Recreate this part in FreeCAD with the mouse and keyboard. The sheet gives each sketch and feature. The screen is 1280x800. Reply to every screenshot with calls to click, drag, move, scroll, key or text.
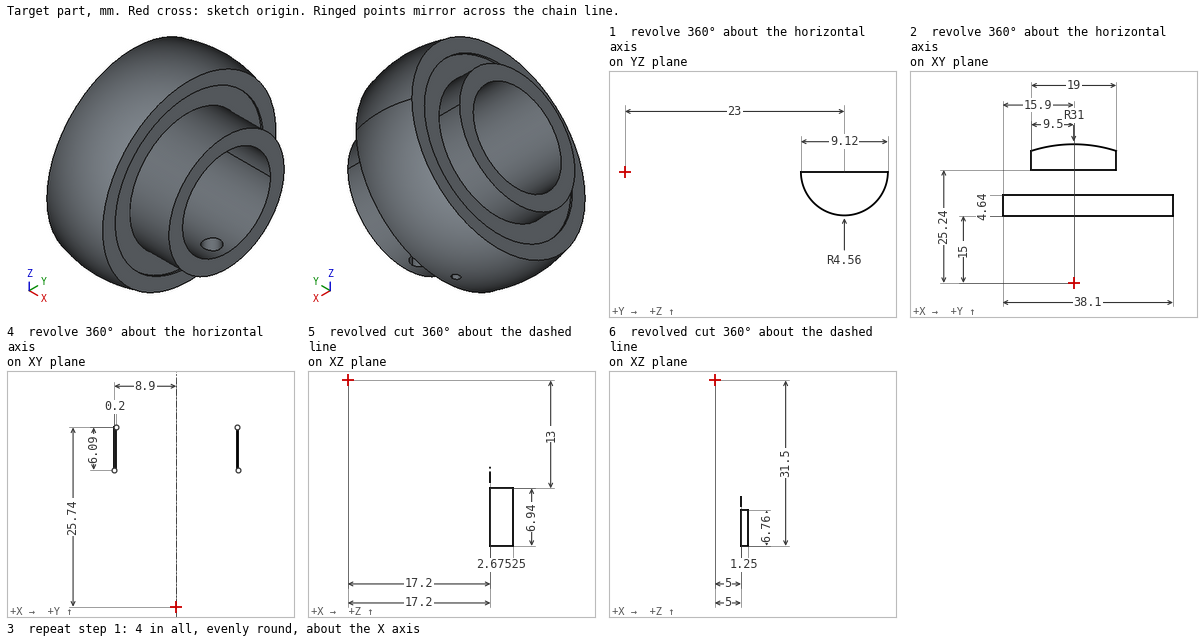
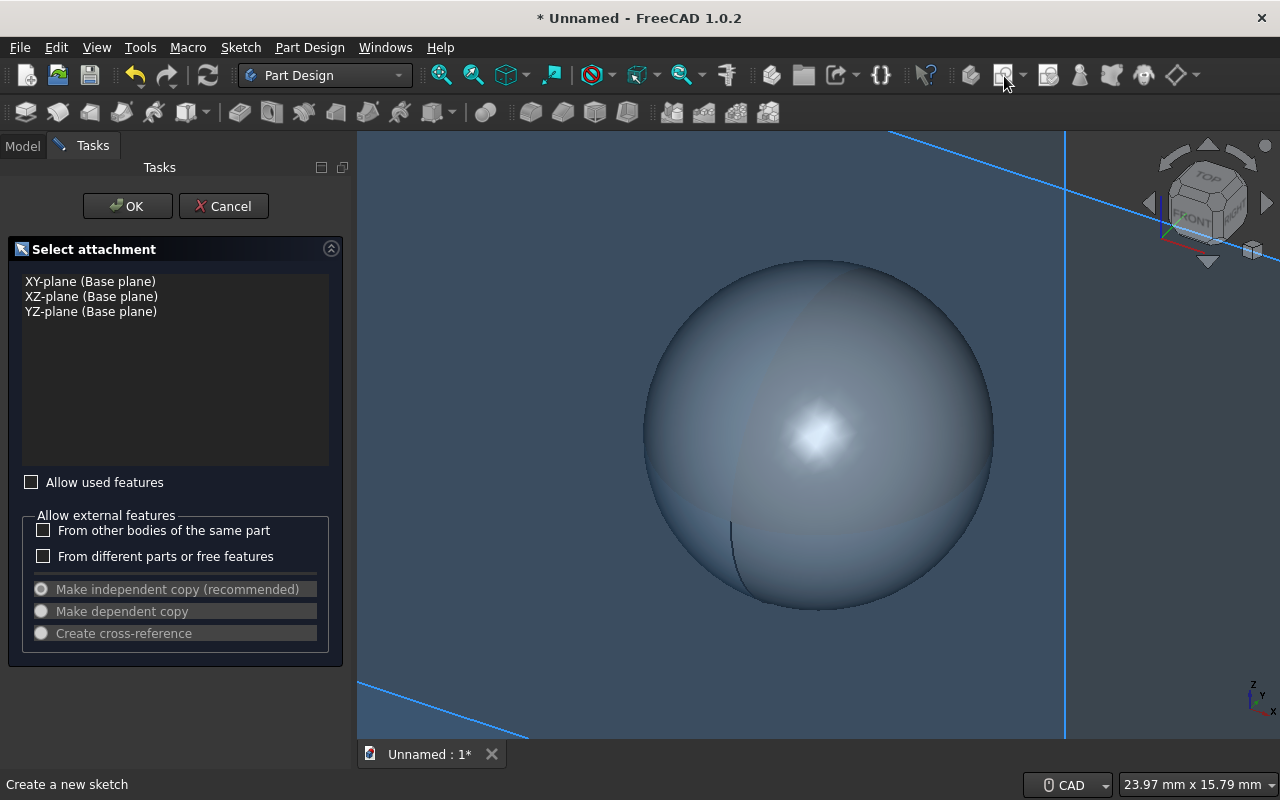
click(82, 282)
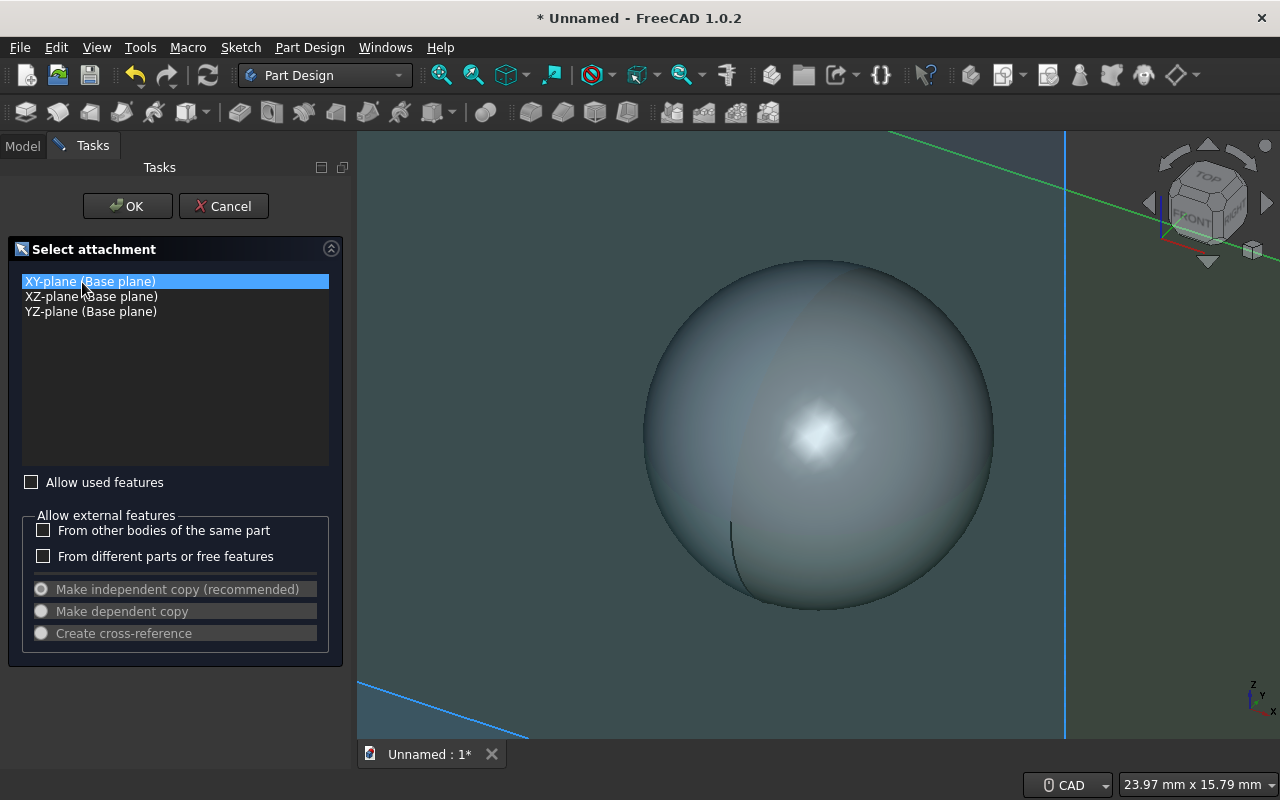
click(128, 206)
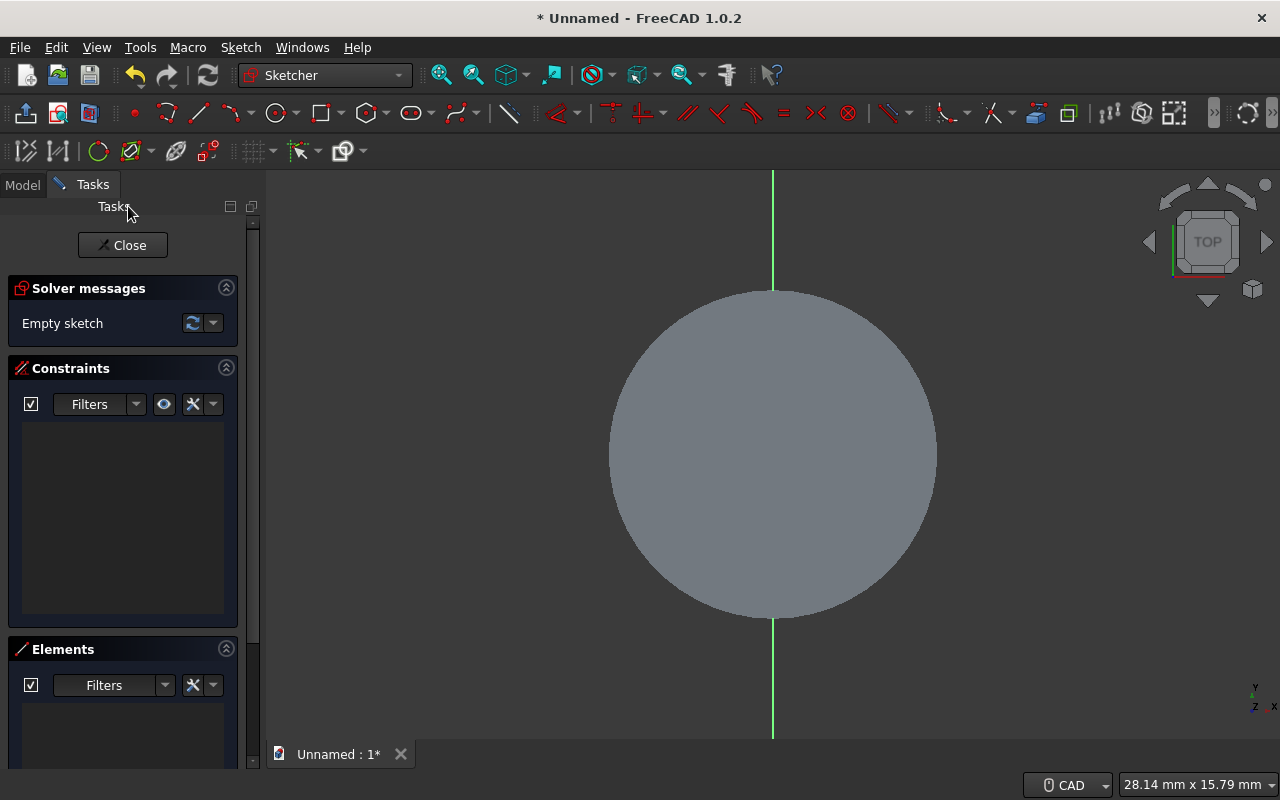
key(q)
key(s)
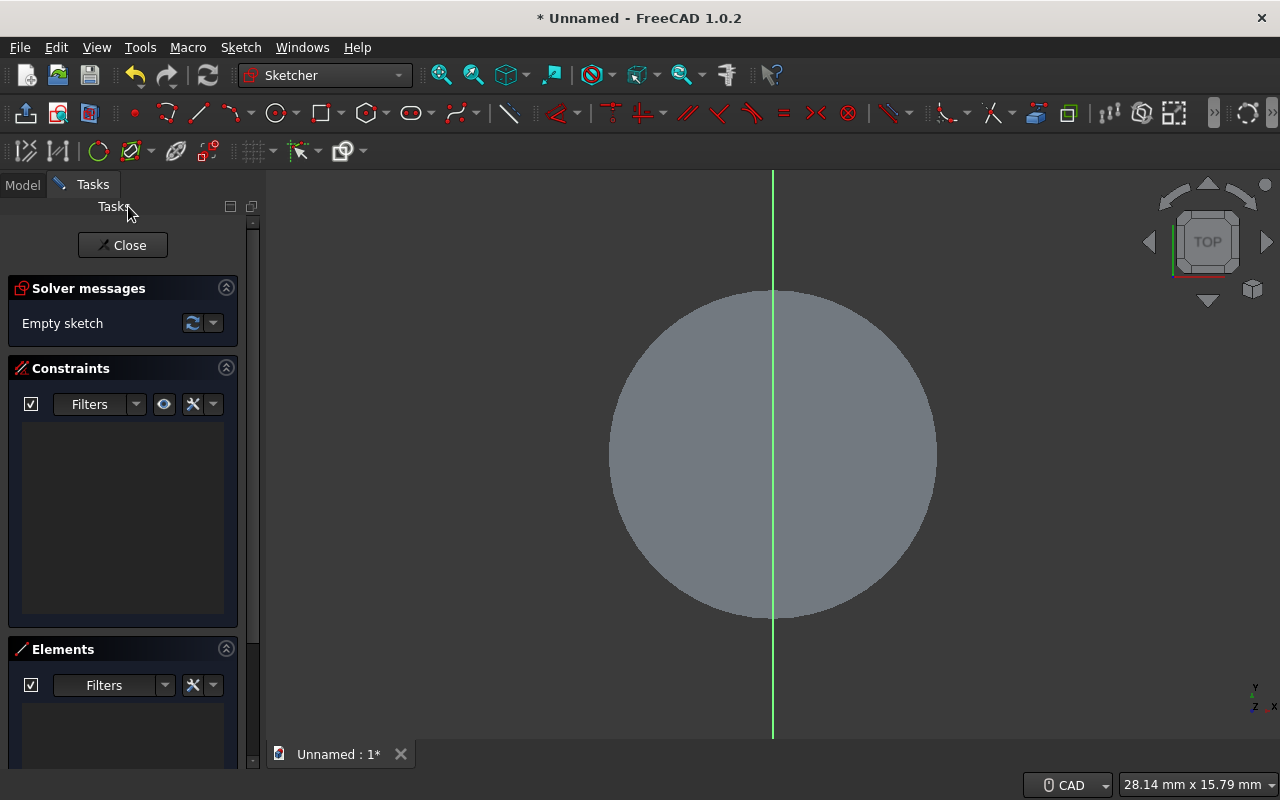
scroll(626, 338, down, 6)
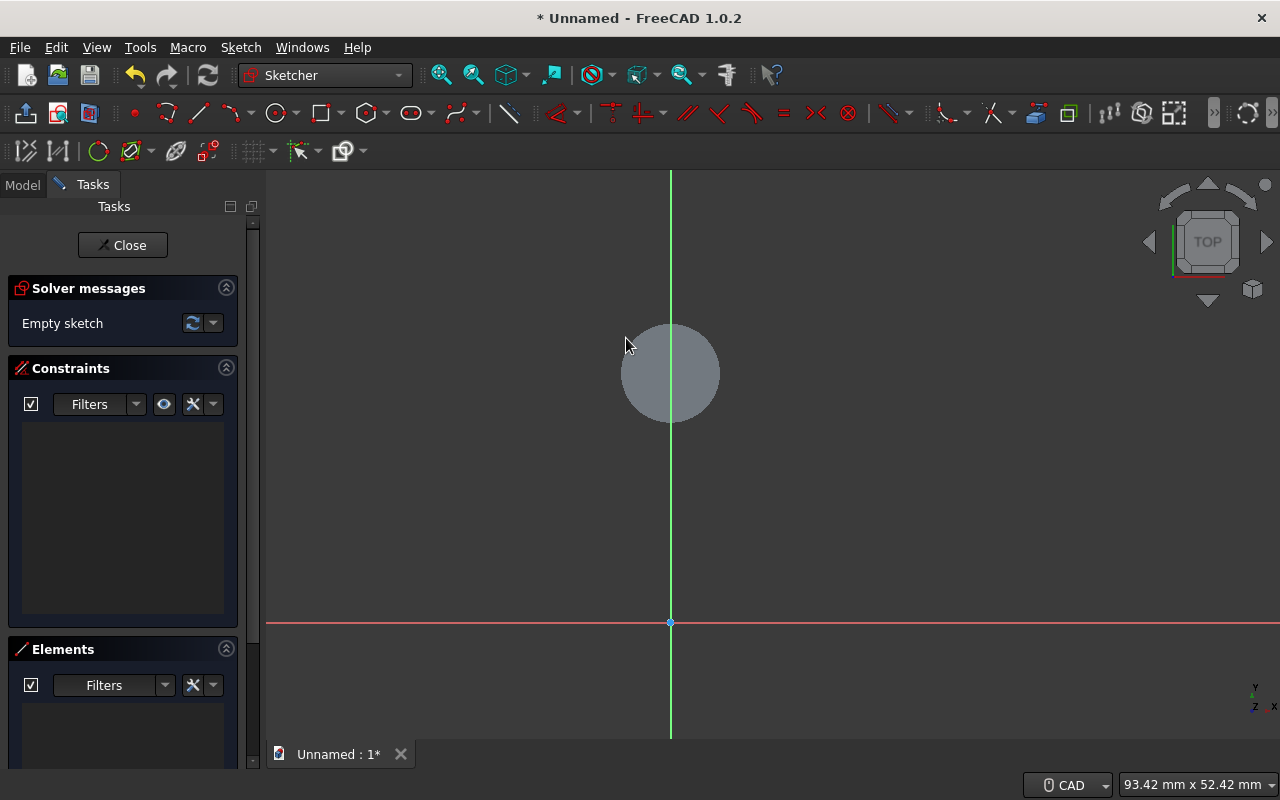
click(168, 114)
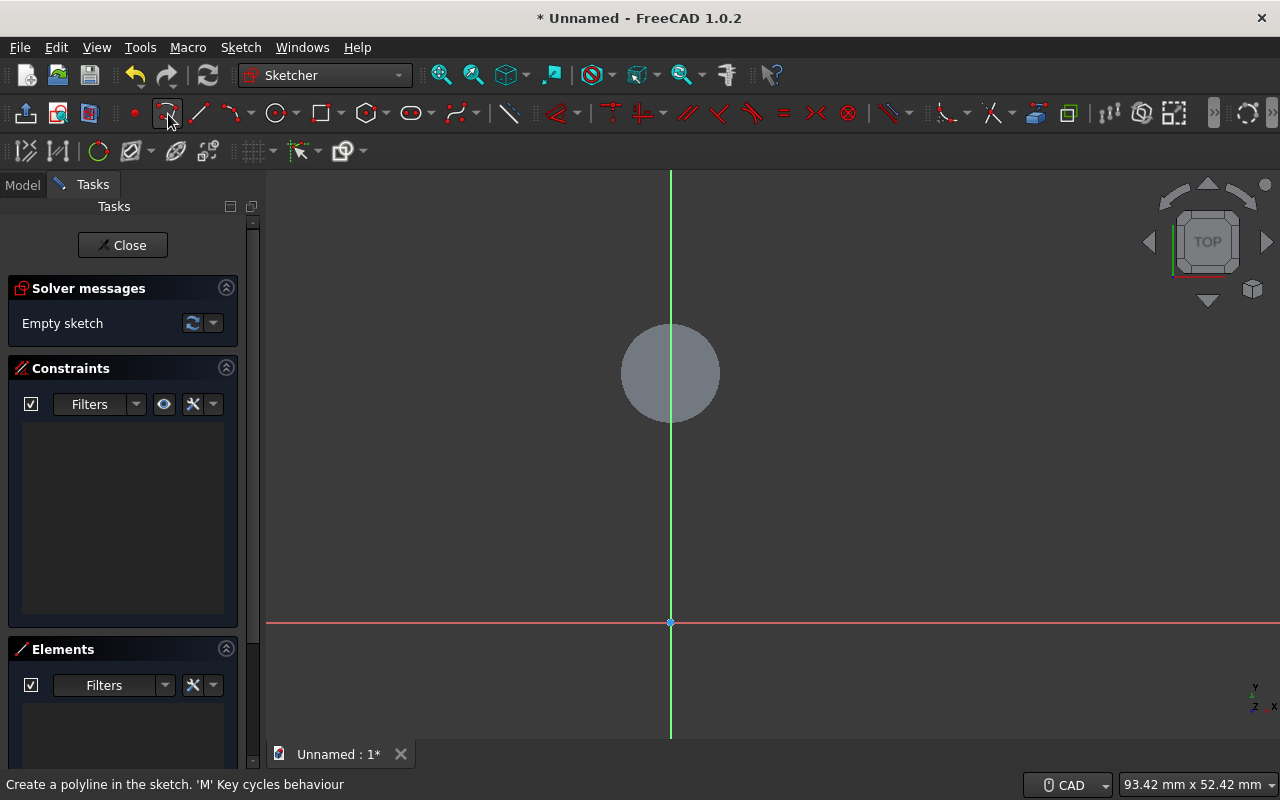
click(567, 303)
click(567, 349)
click(774, 349)
click(774, 303)
right_click(774, 303)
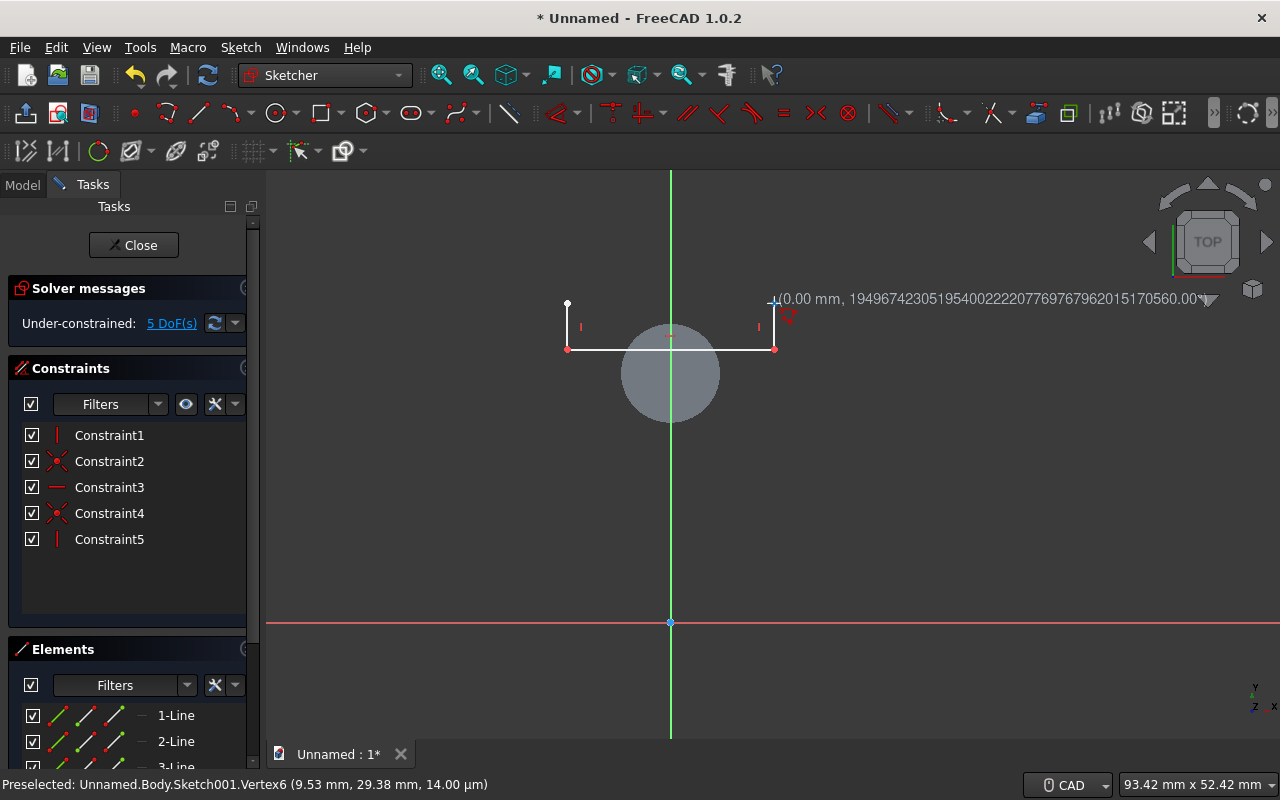
key(g)
key(3)
key(a)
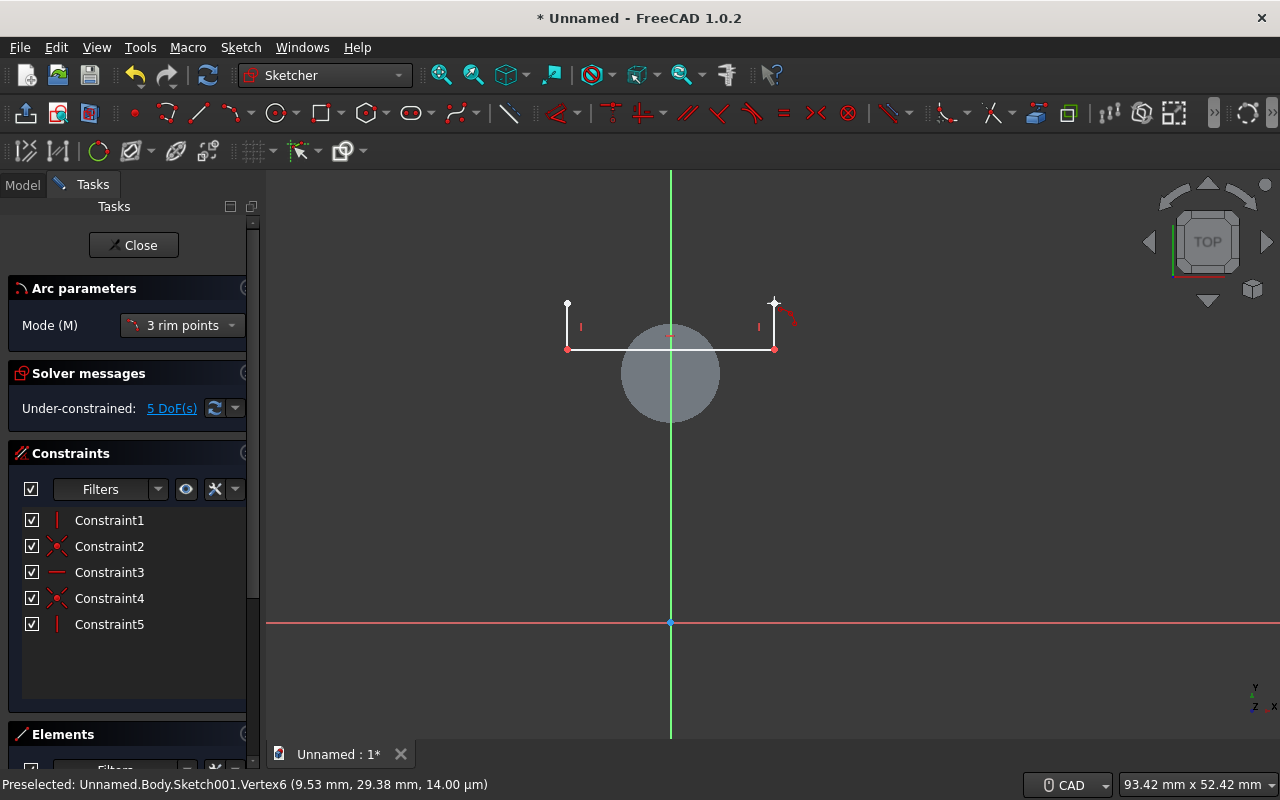
click(774, 304)
click(567, 304)
click(691, 287)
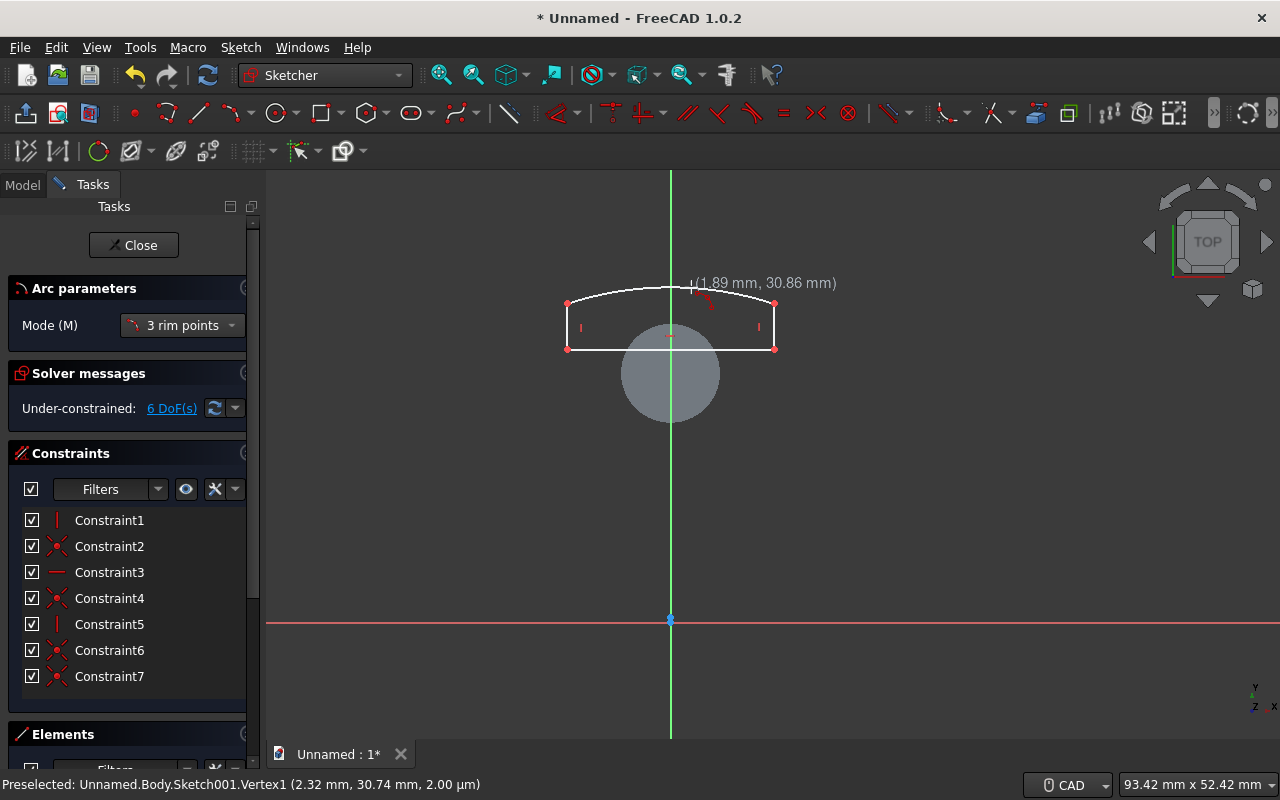
click(322, 114)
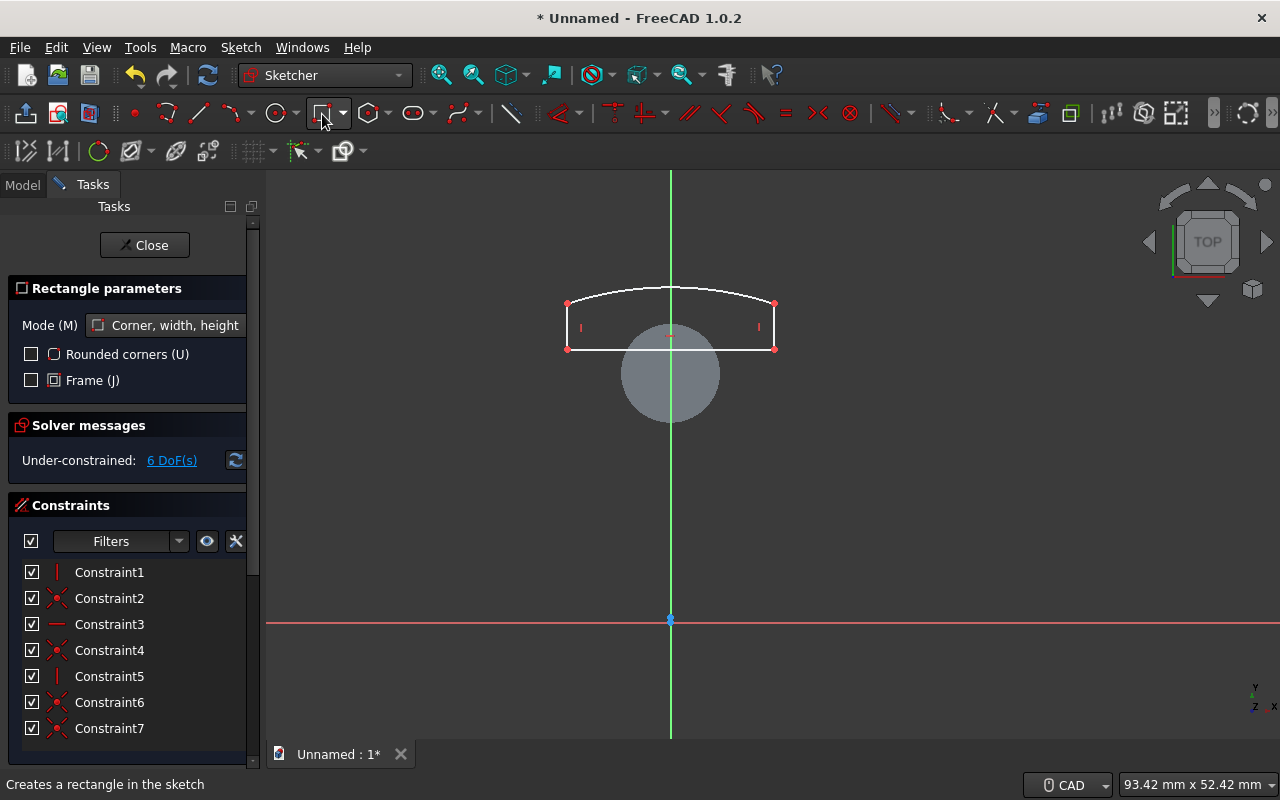
click(498, 410)
click(911, 460)
key(Escape)